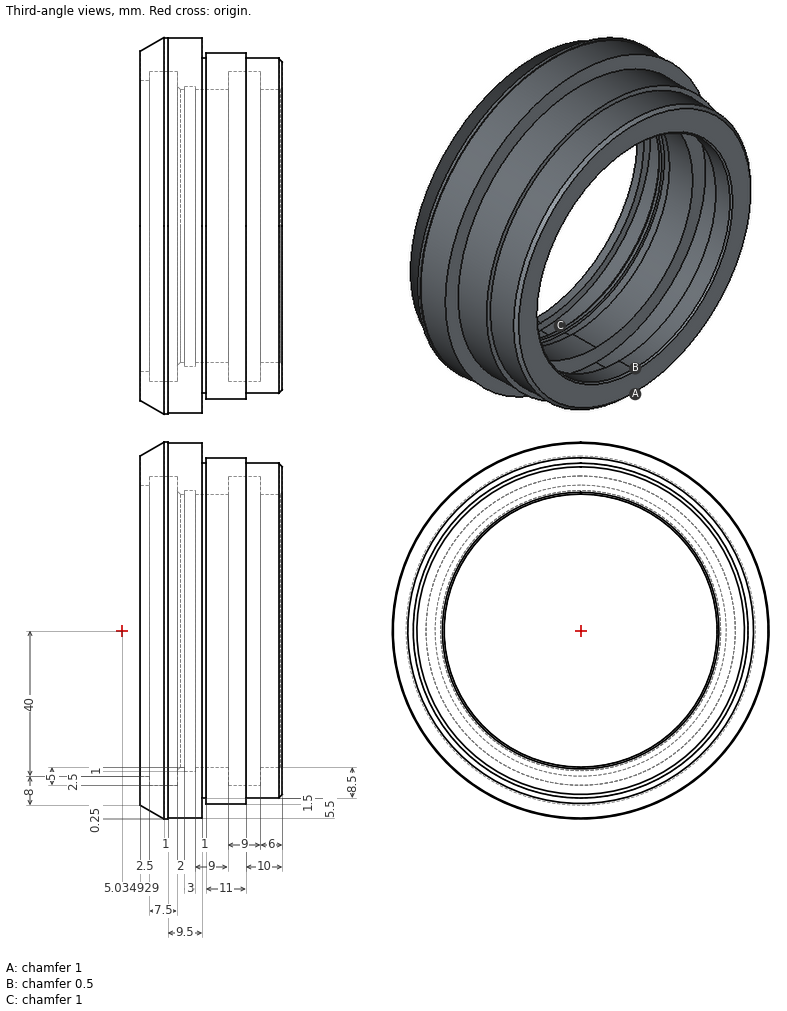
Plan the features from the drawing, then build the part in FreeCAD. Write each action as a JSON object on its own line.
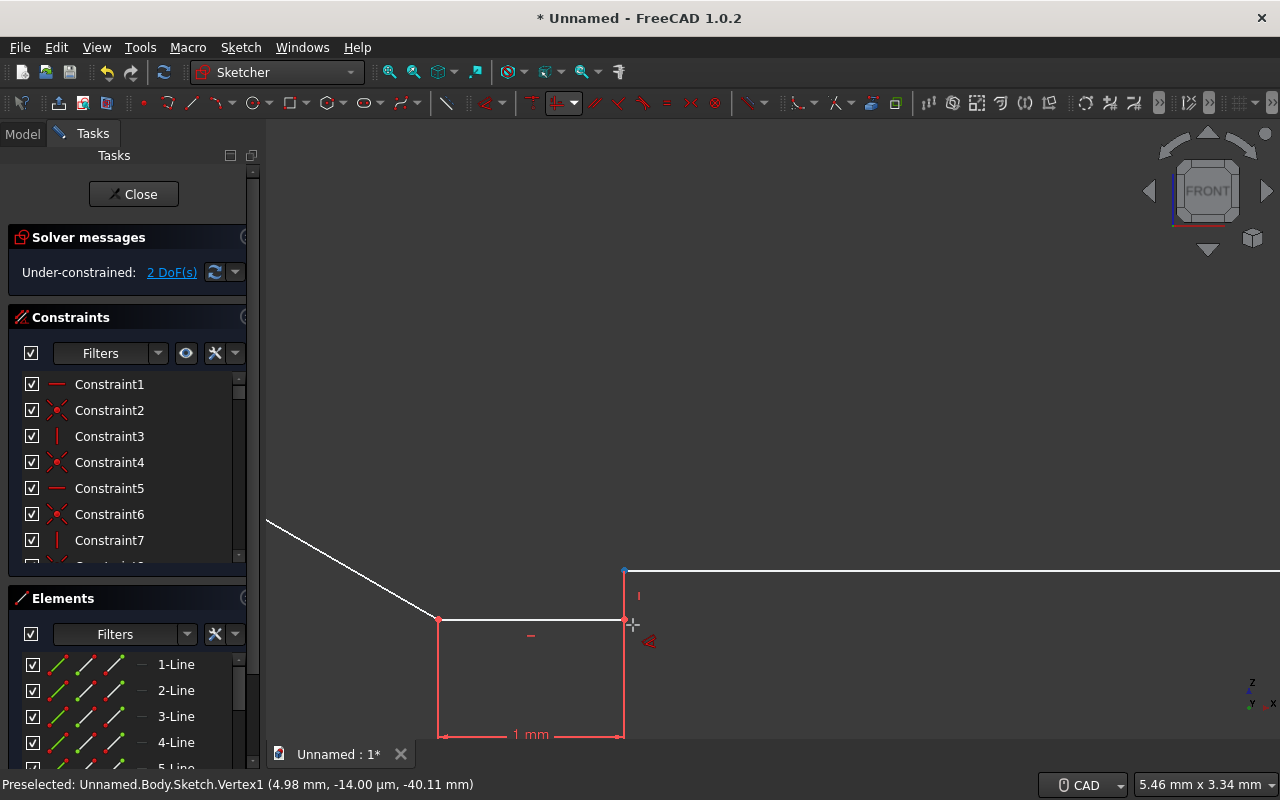
{"action": "left_click", "coordinate": [624, 595]}
{"action": "left_click", "coordinate": [590, 595]}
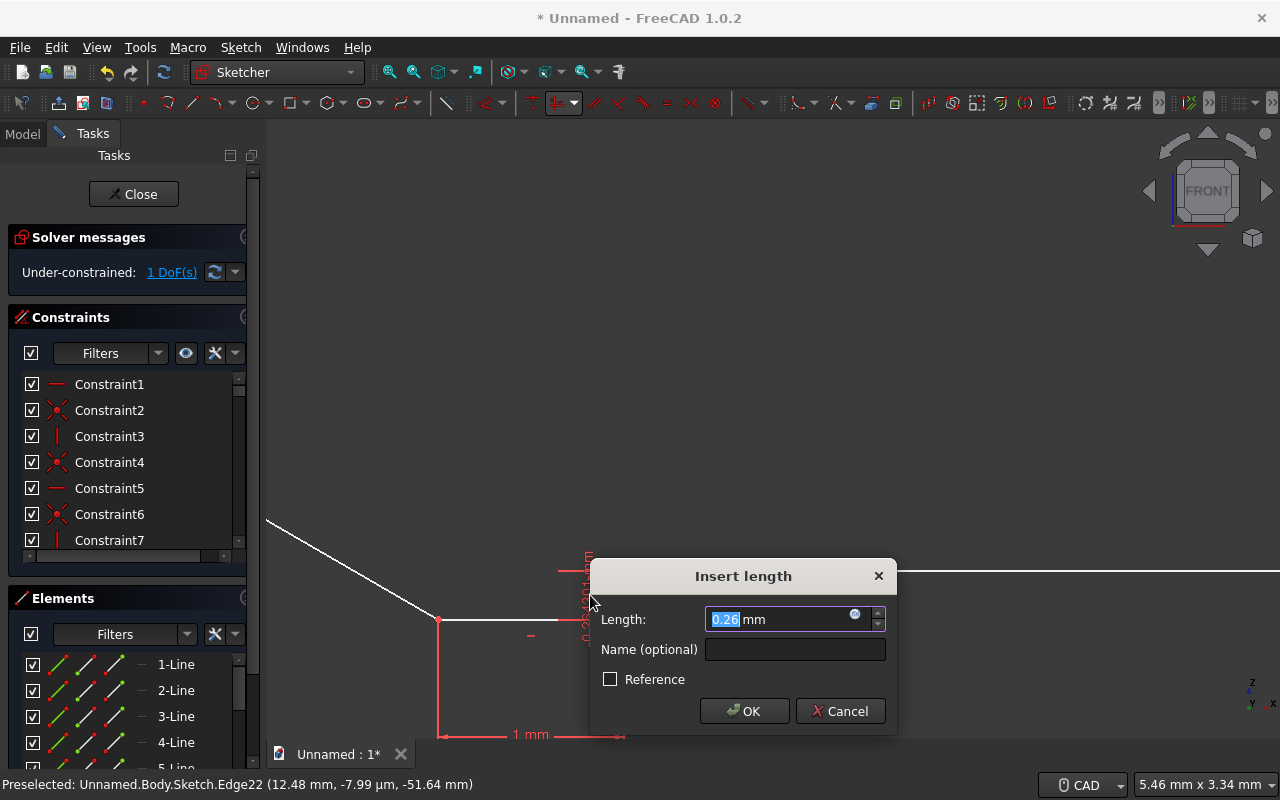
{"action": "type", "text": "0.25"}
{"action": "key", "text": "Return"}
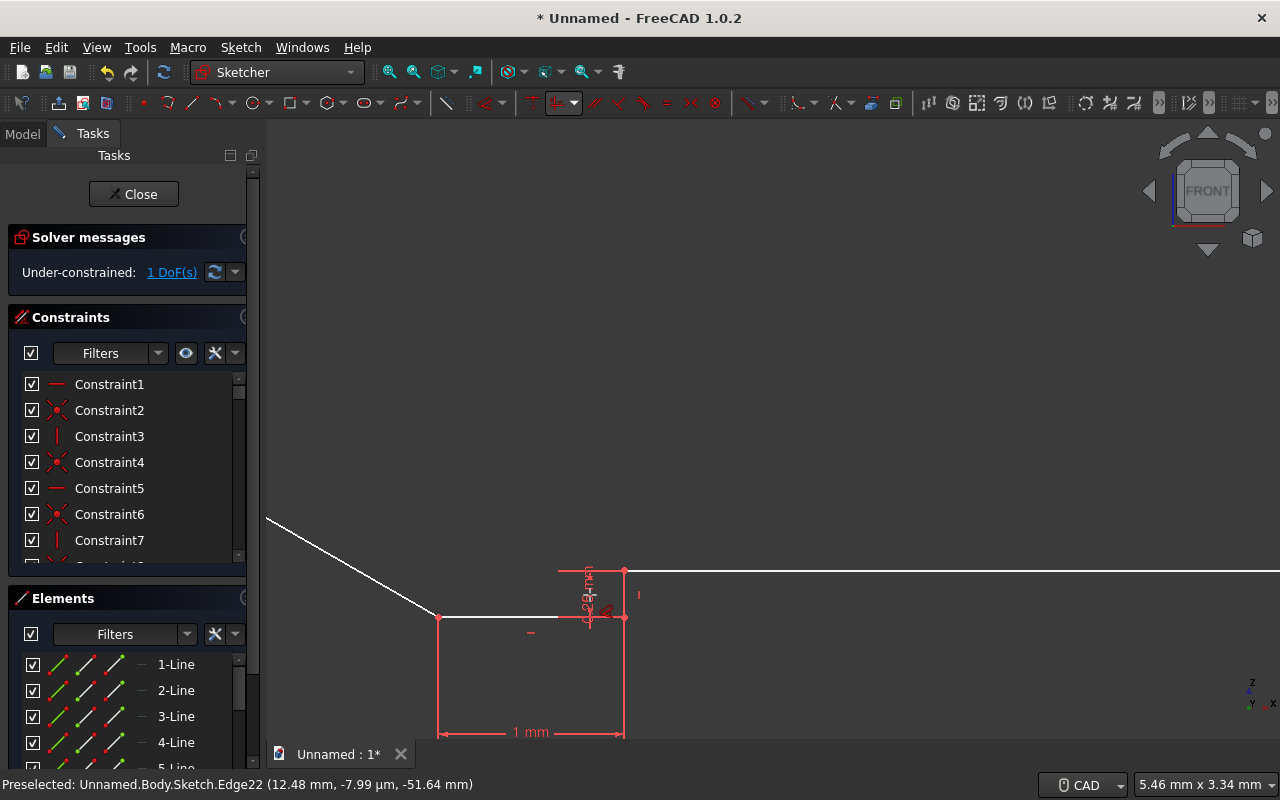
{"action": "scroll", "coordinate": [616, 671], "scroll_direction": "down", "scroll_amount": 15}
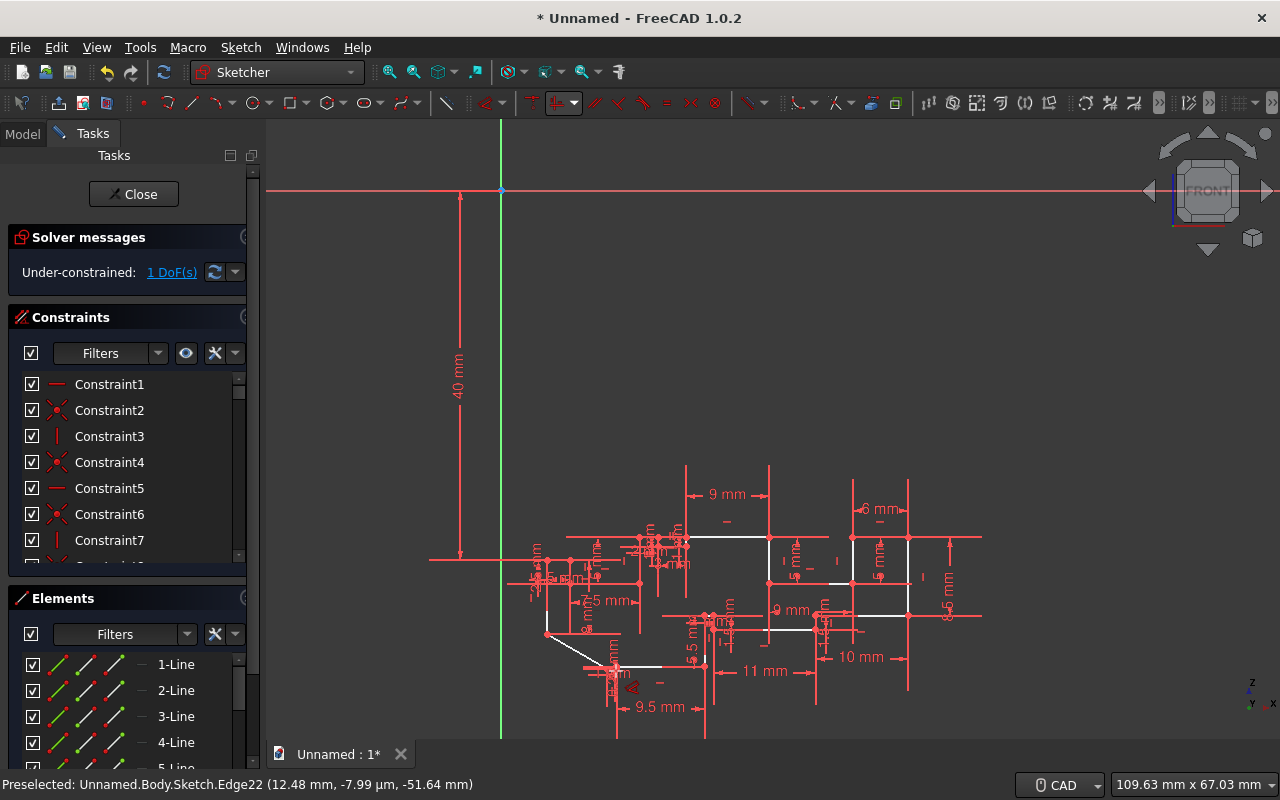
{"action": "left_click", "coordinate": [547, 560]}
{"action": "left_click", "coordinate": [524, 157]}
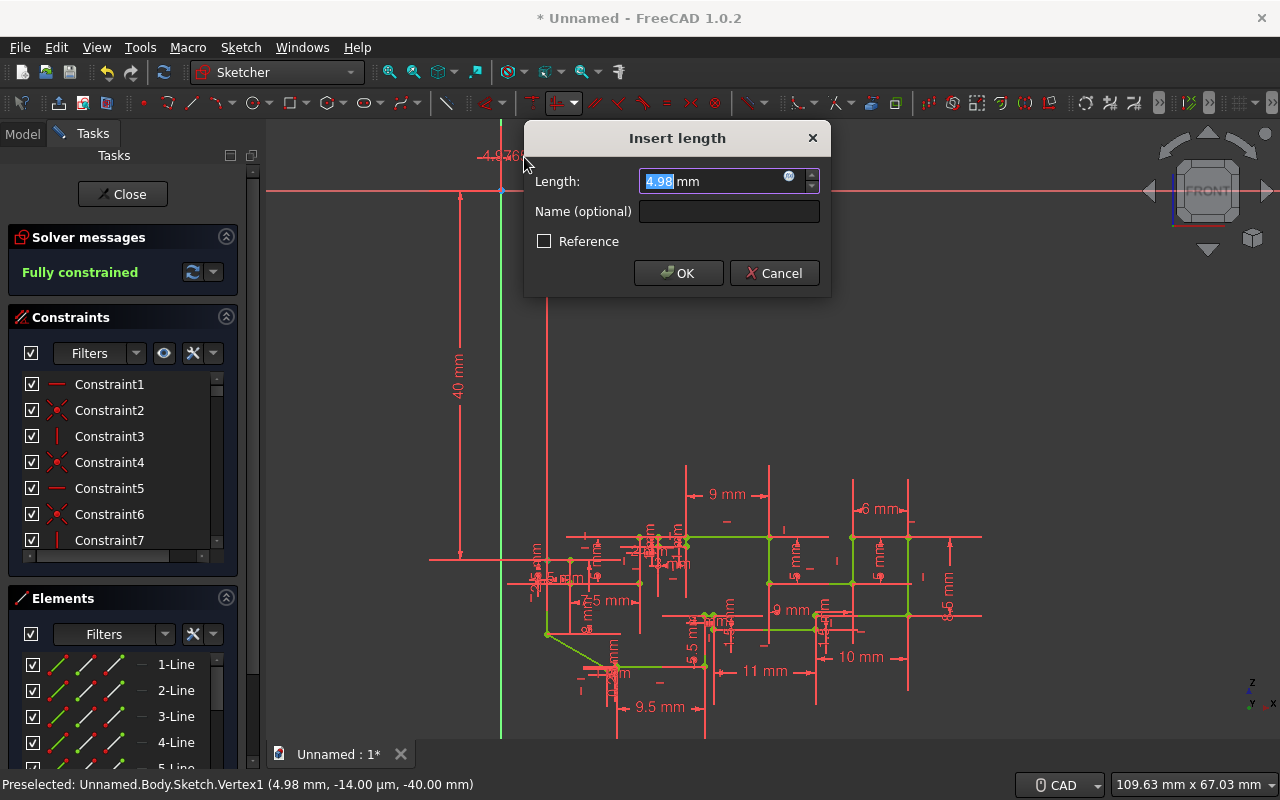
{"action": "type", "text": "5.034929"}
{"action": "key", "text": "Return"}
{"action": "key", "text": "Escape"}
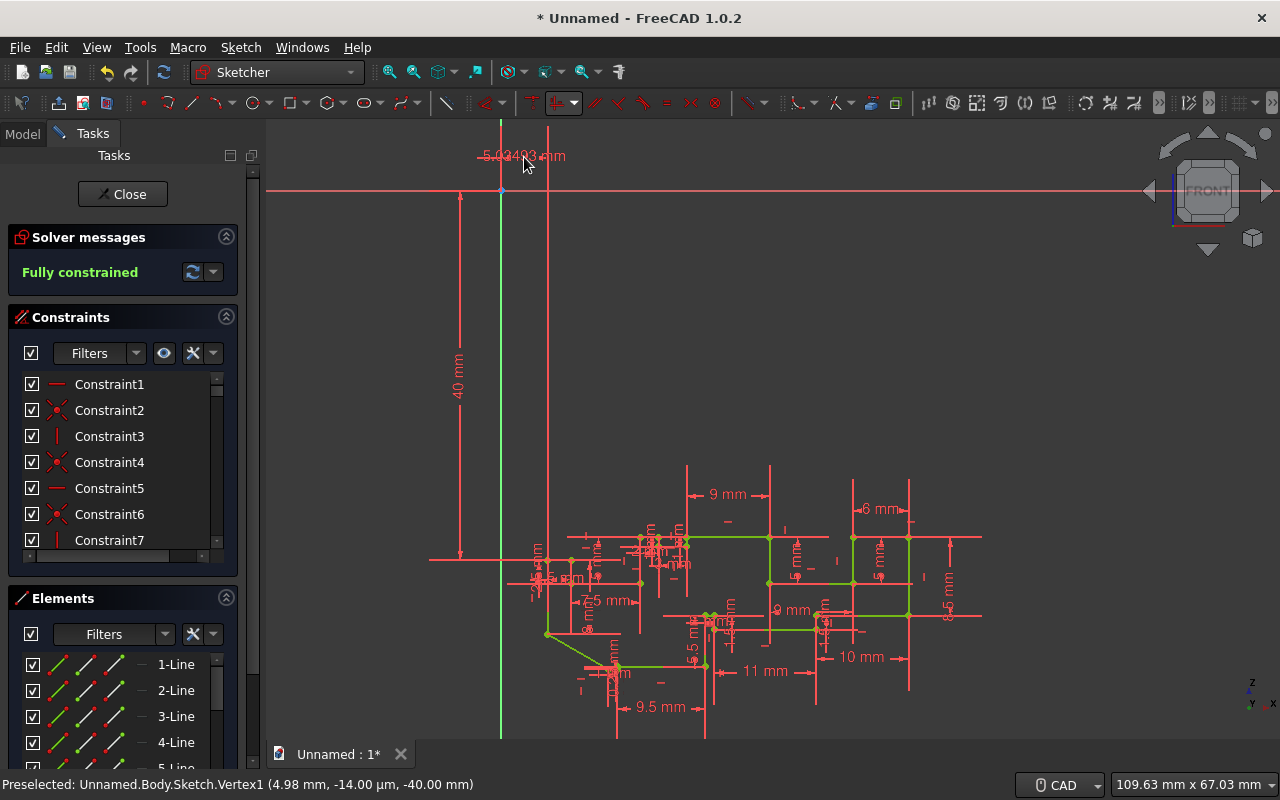
{"action": "left_click", "coordinate": [123, 194]}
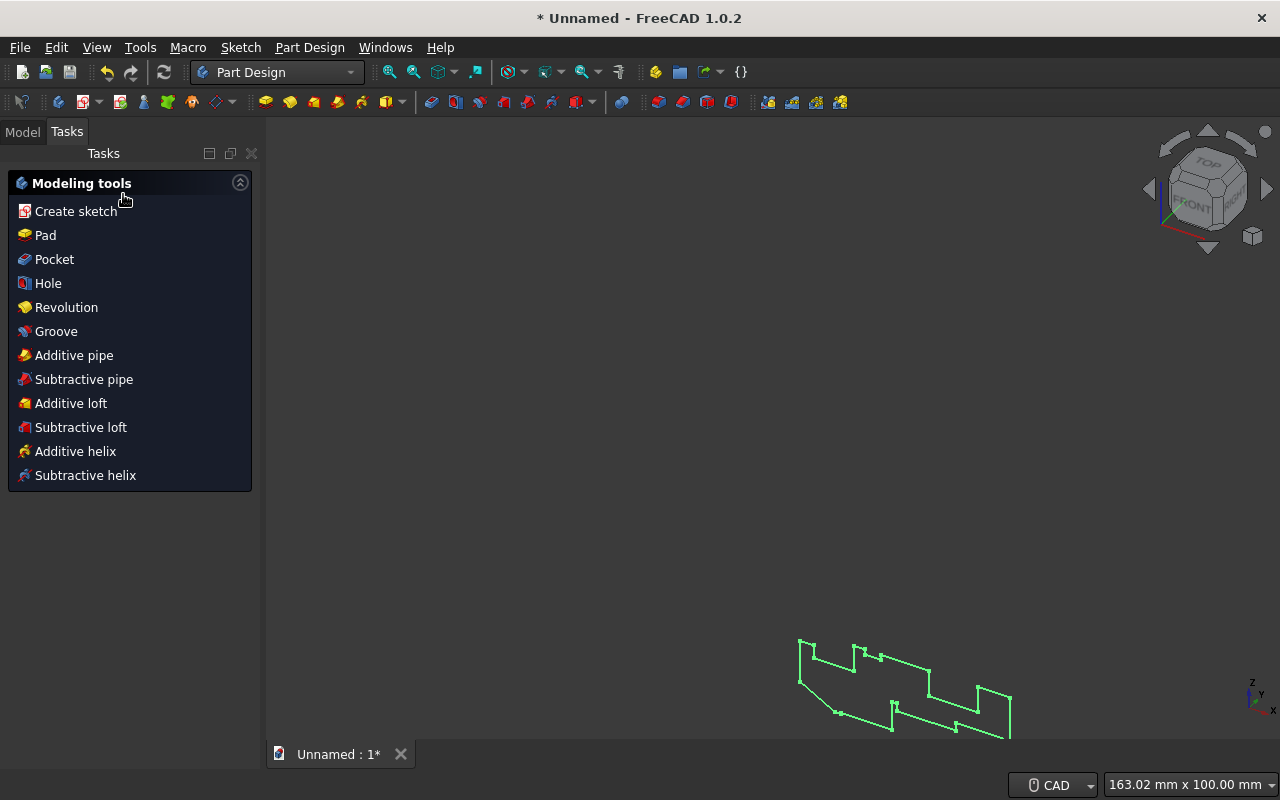
{"action": "left_click", "coordinate": [290, 102]}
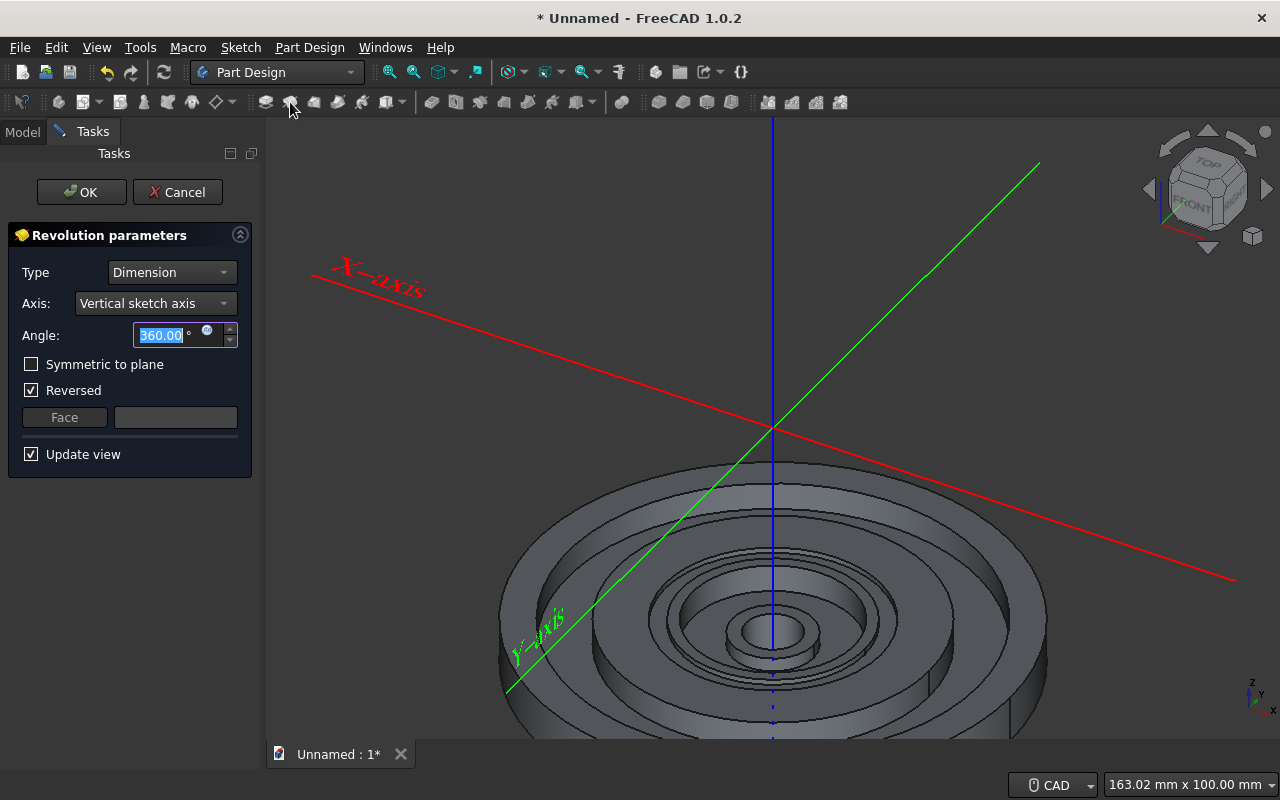
{"action": "left_click", "coordinate": [156, 304]}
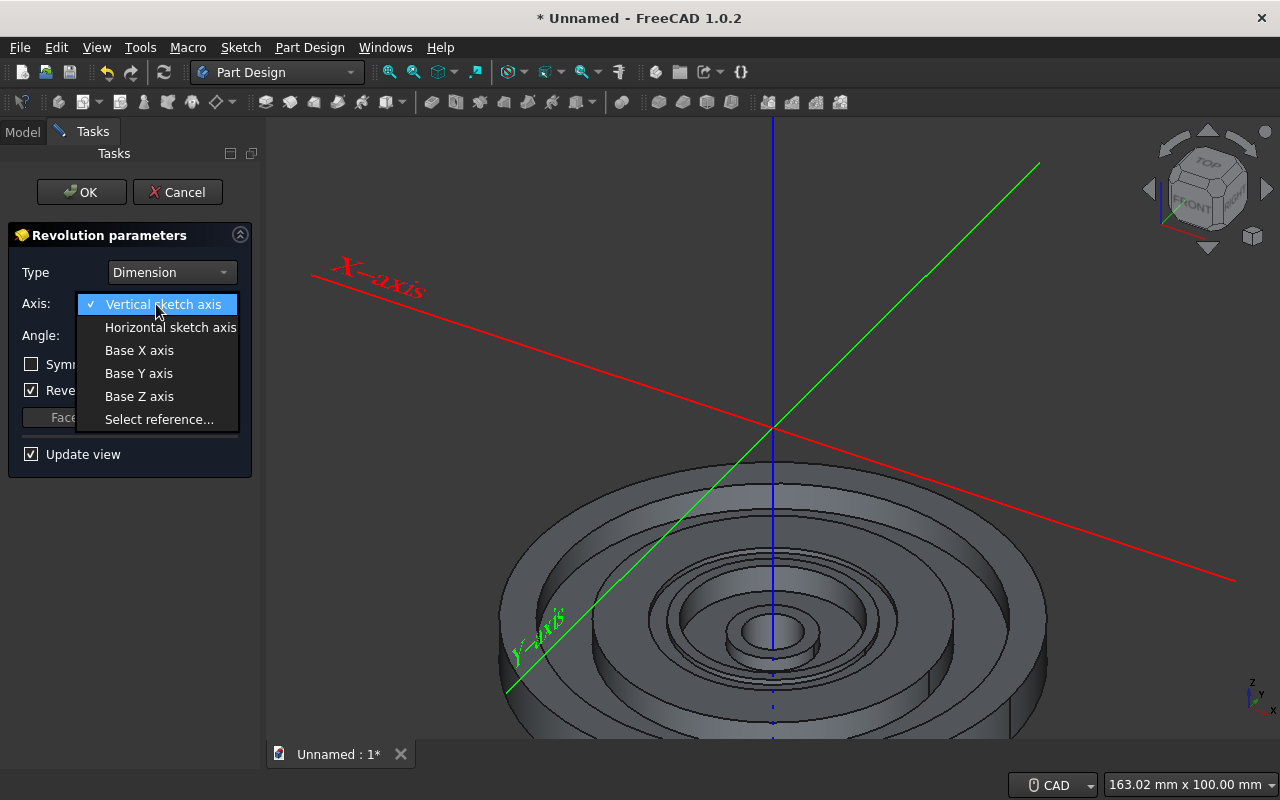
{"action": "left_click", "coordinate": [156, 328]}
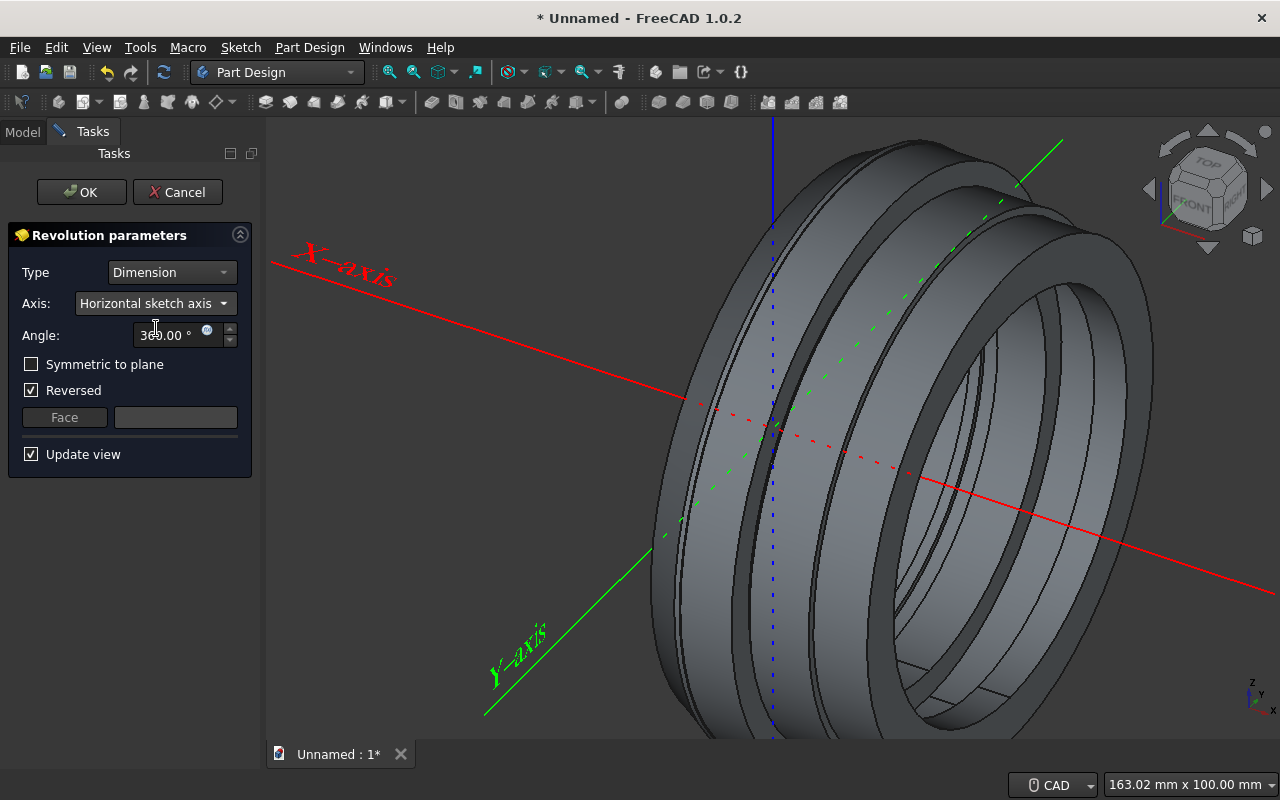
{"action": "left_click", "coordinate": [82, 192]}